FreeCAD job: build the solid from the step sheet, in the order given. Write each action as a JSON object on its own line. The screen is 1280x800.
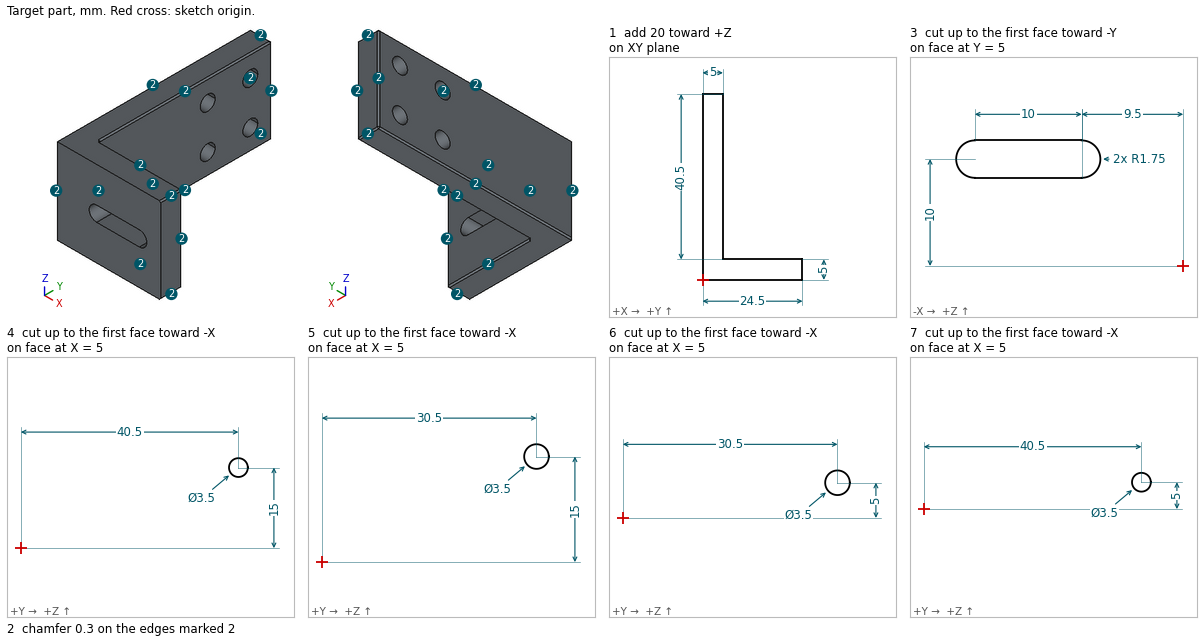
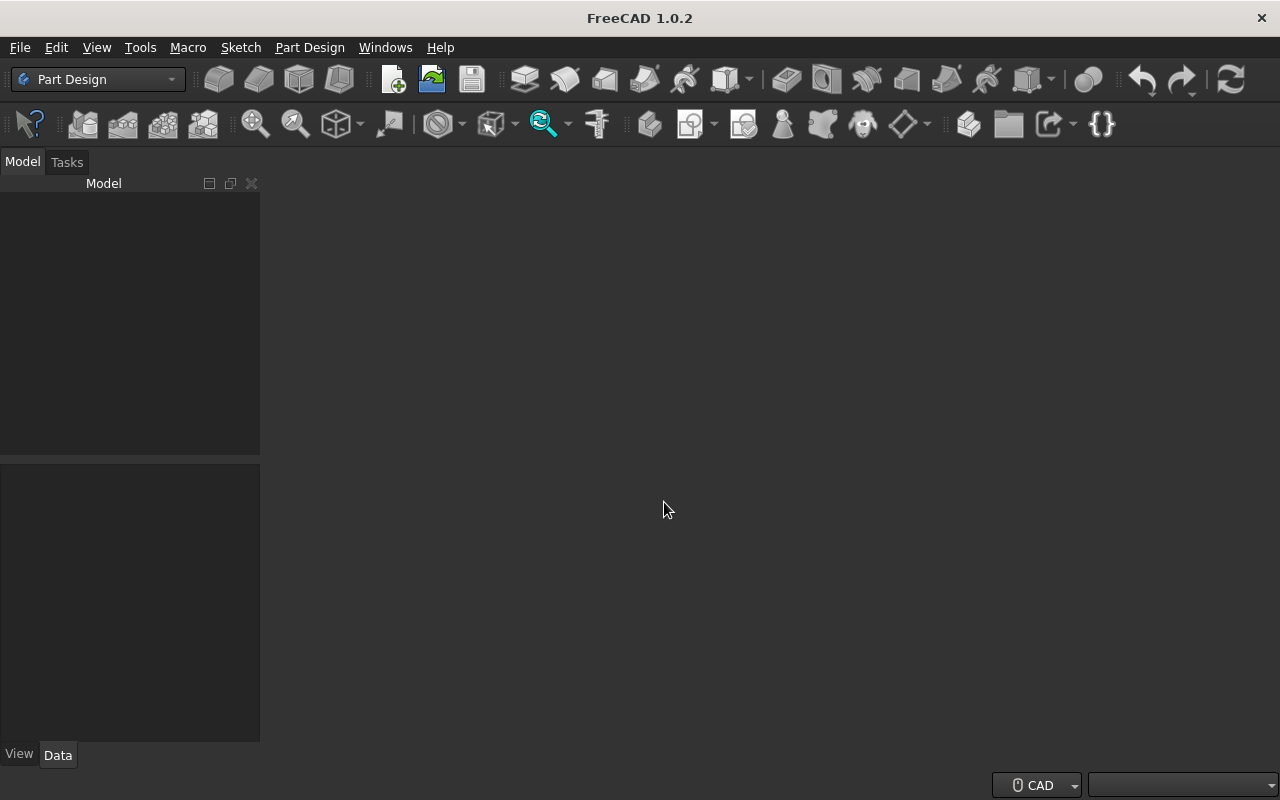
{"action": "left_click", "coordinate": [392, 80]}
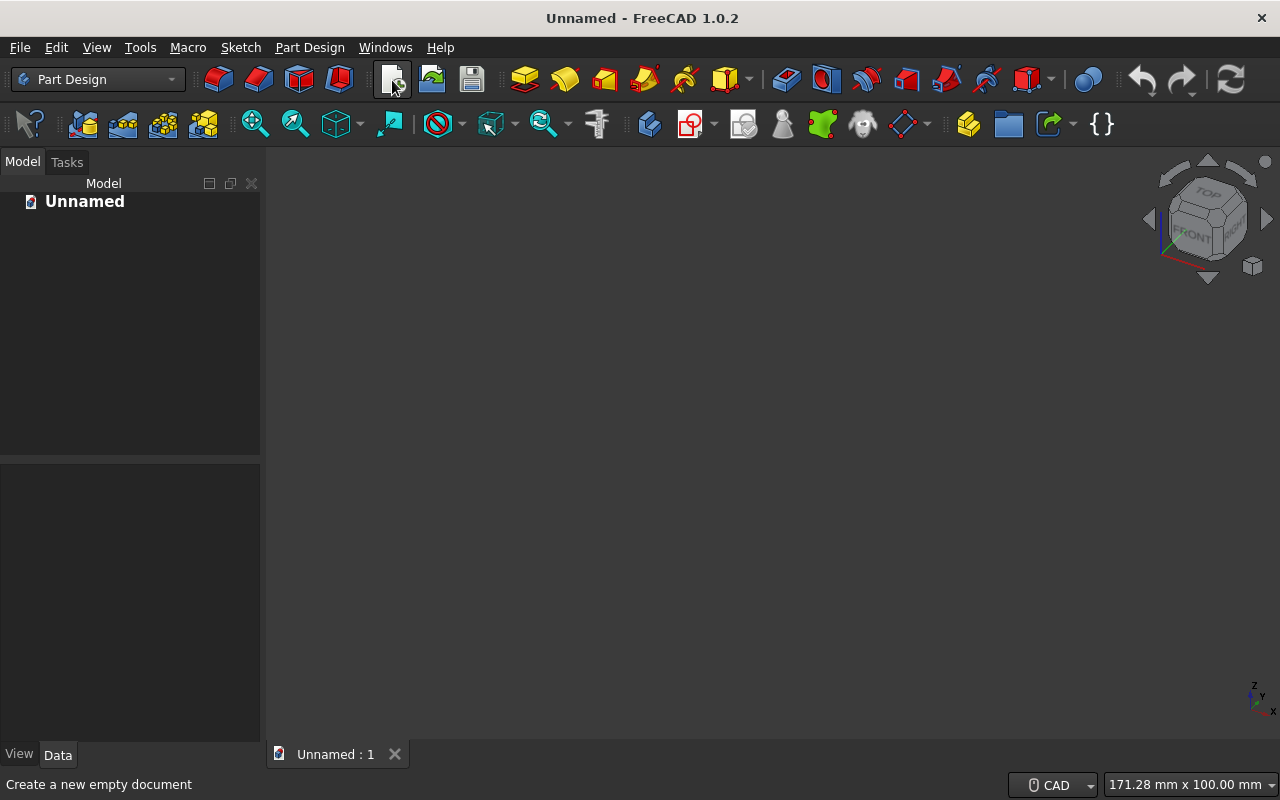
{"action": "left_click", "coordinate": [690, 124]}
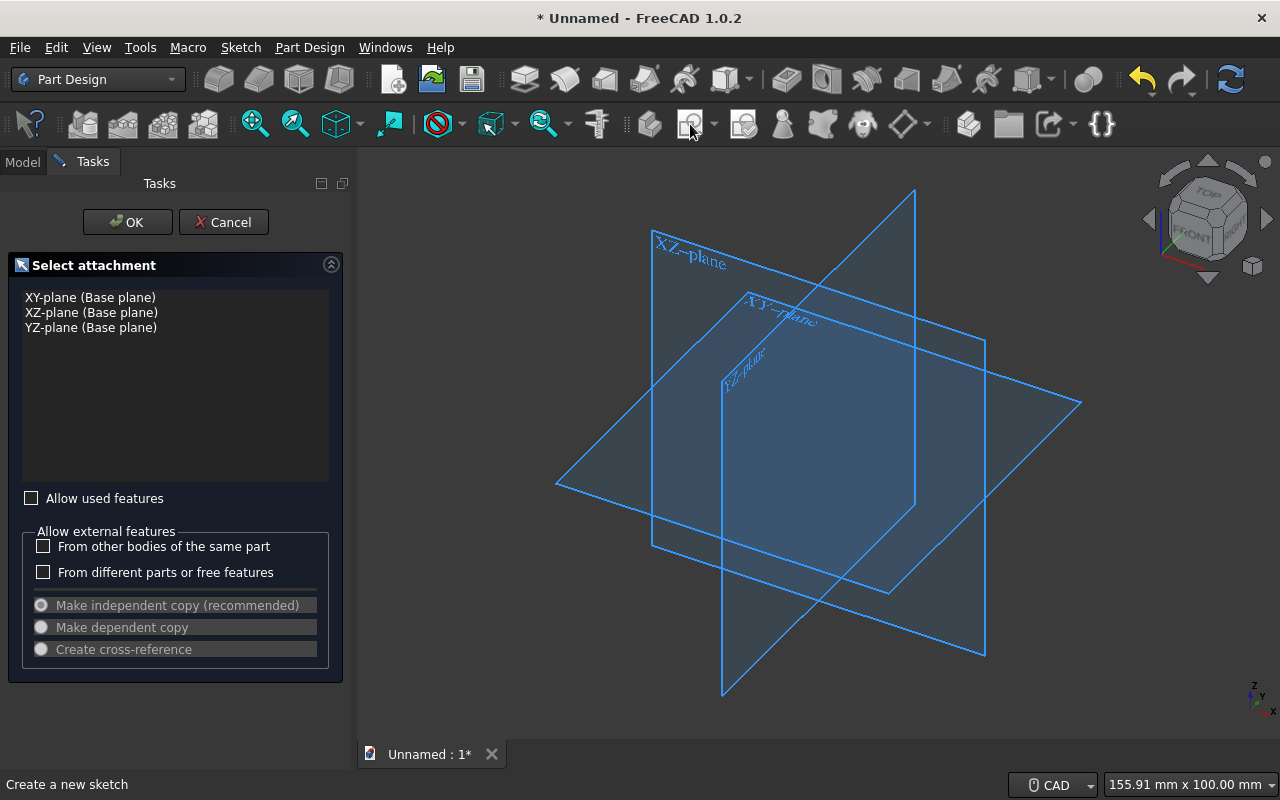
{"action": "left_click", "coordinate": [82, 298]}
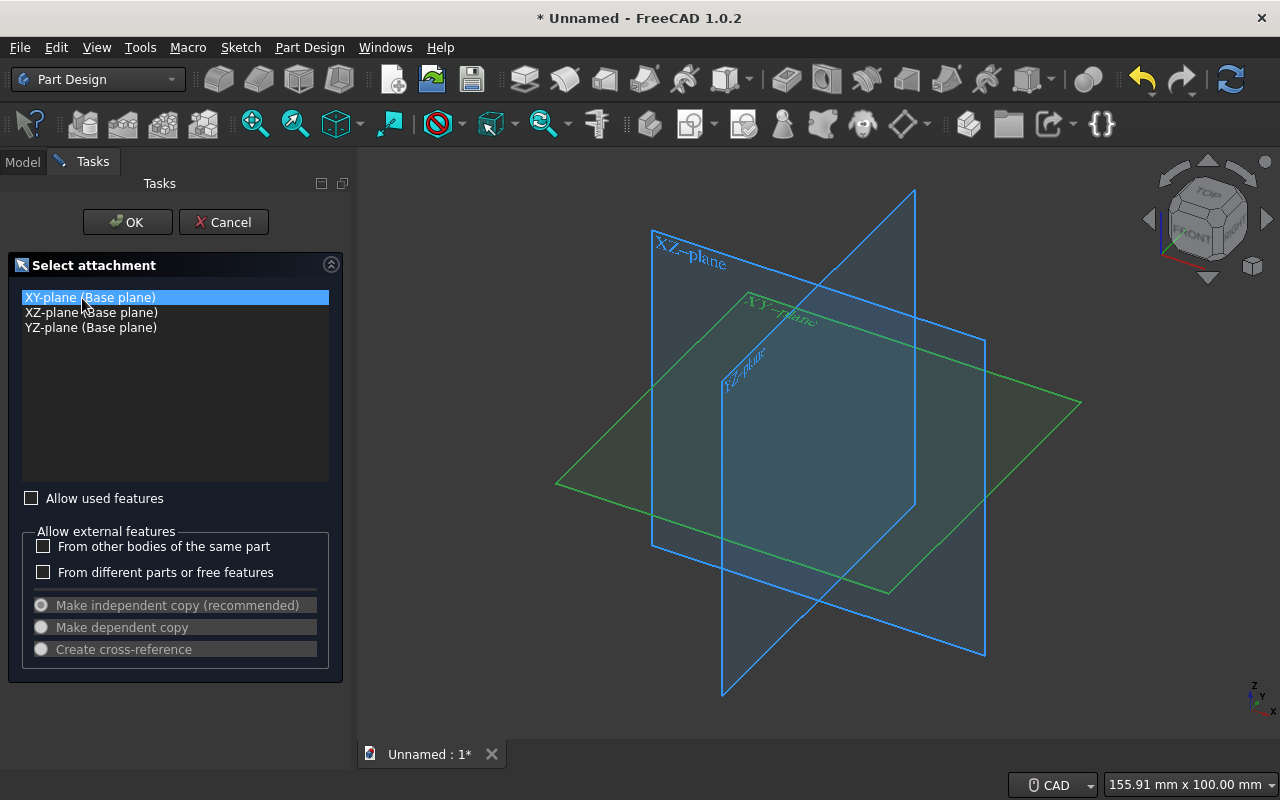
{"action": "left_click", "coordinate": [128, 222]}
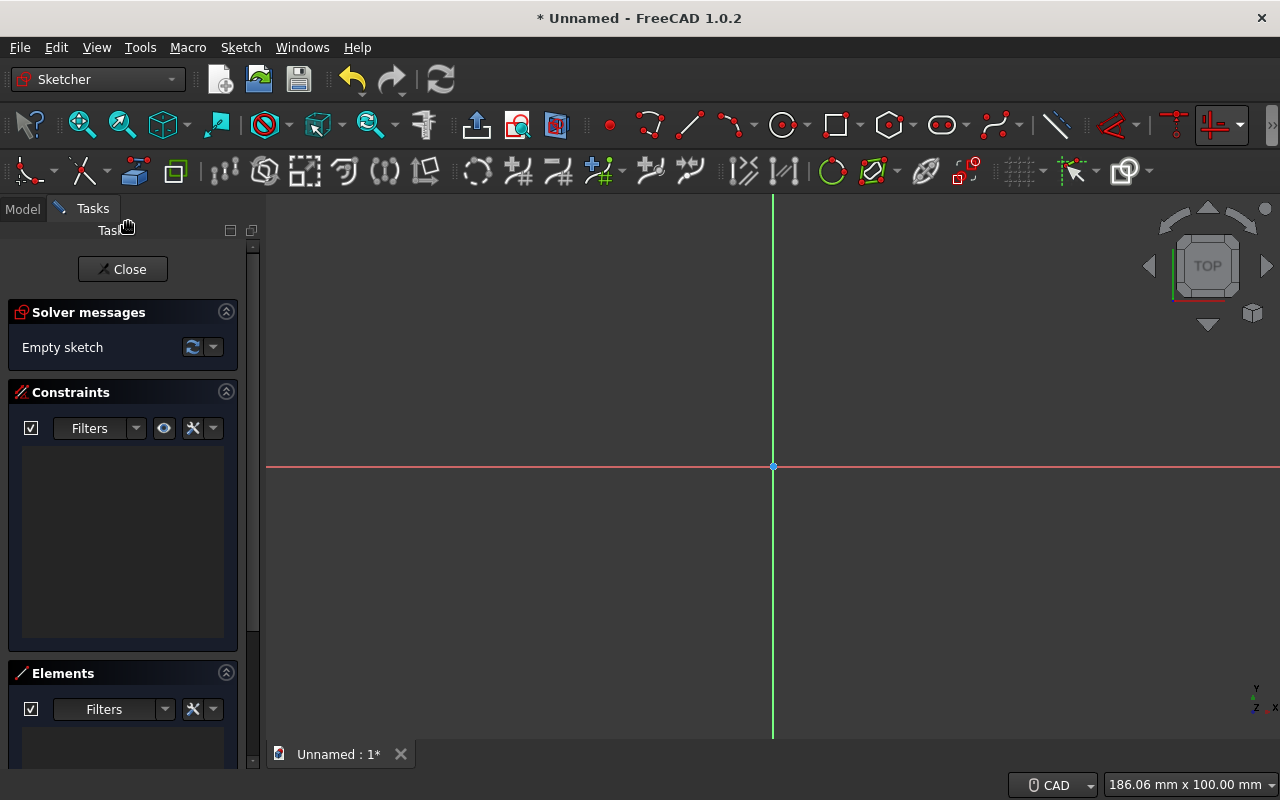
{"action": "scroll", "coordinate": [294, 711], "scroll_direction": "down", "scroll_amount": 1}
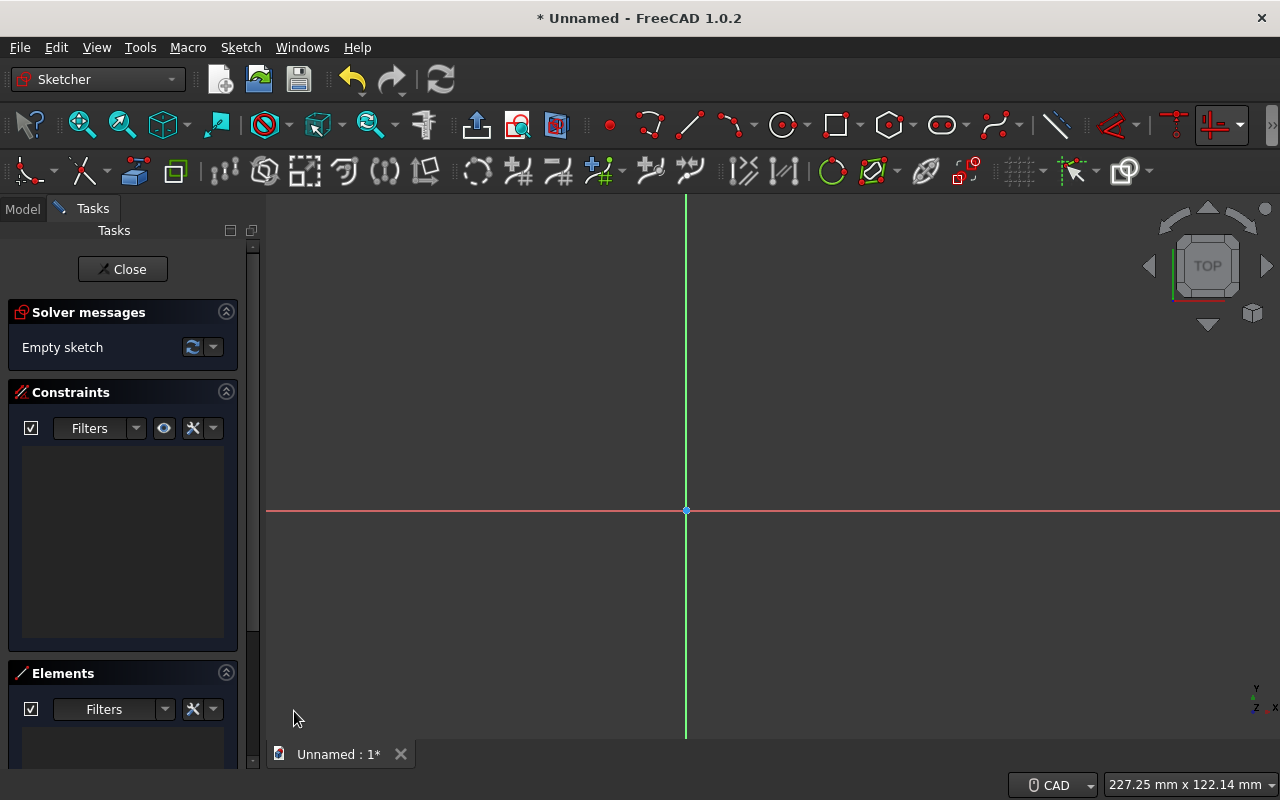
{"action": "scroll", "coordinate": [785, 340], "scroll_direction": "up", "scroll_amount": 3}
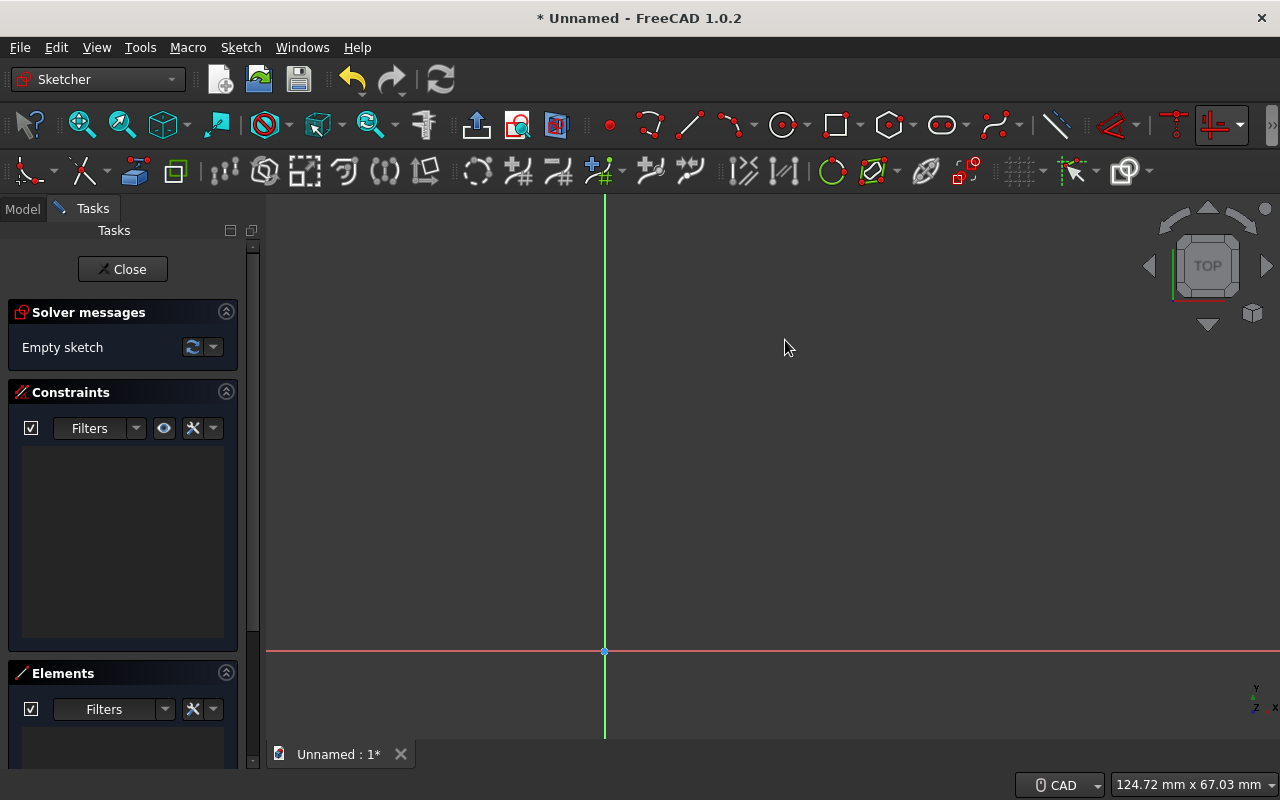
{"action": "key", "text": "g m"}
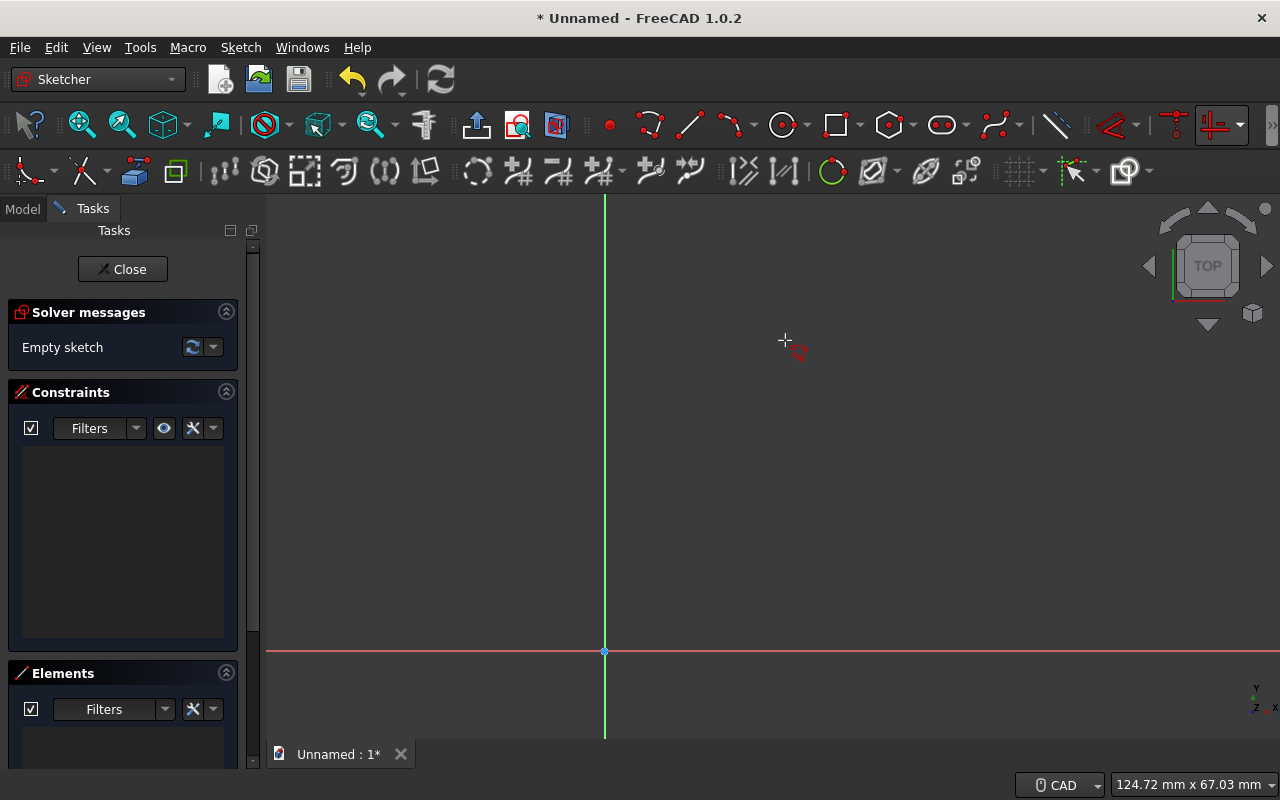
{"action": "left_click", "coordinate": [605, 651]}
{"action": "left_click", "coordinate": [804, 642]}
{"action": "left_click", "coordinate": [804, 611]}
{"action": "left_click", "coordinate": [645, 611]}
{"action": "left_click", "coordinate": [645, 281]}
{"action": "left_click", "coordinate": [614, 281]}
{"action": "left_click", "coordinate": [605, 651]}
{"action": "key", "text": "Escape"}
{"action": "key", "text": "Escape"}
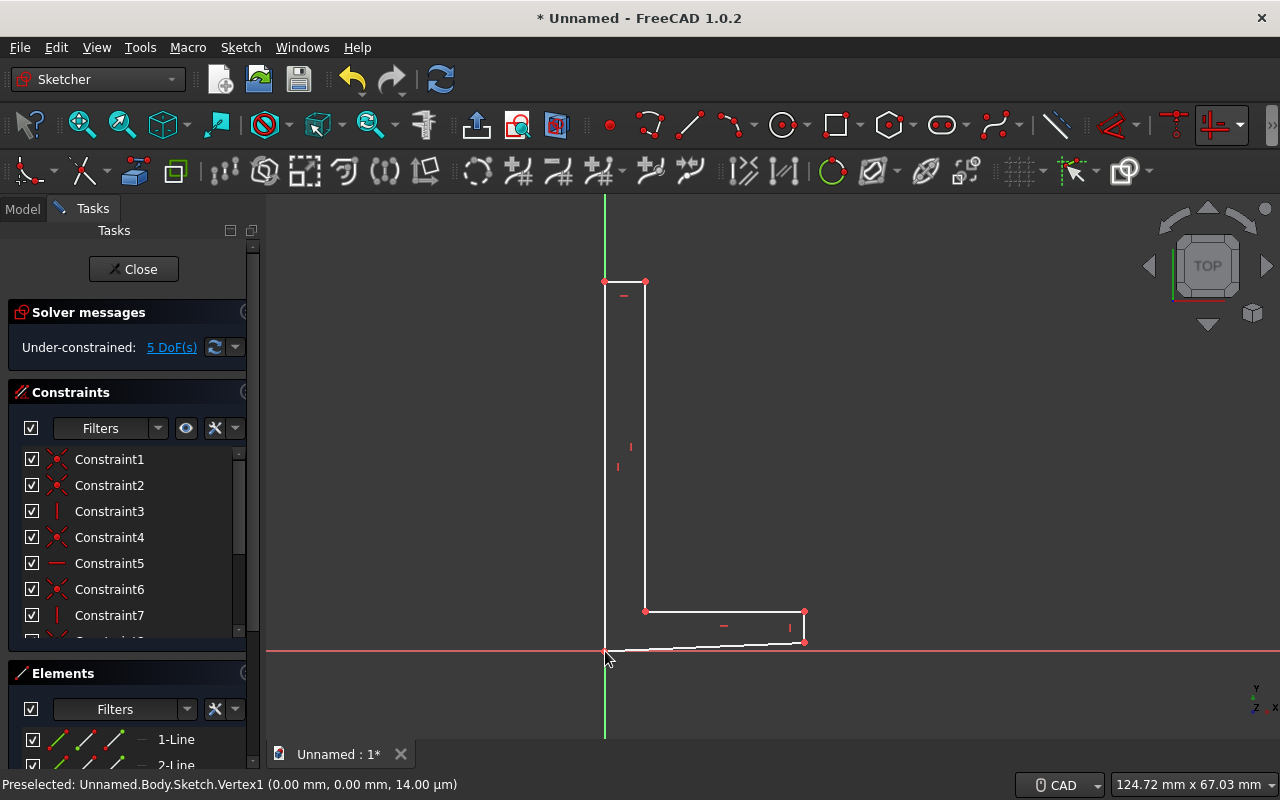
{"action": "left_click", "coordinate": [664, 649]}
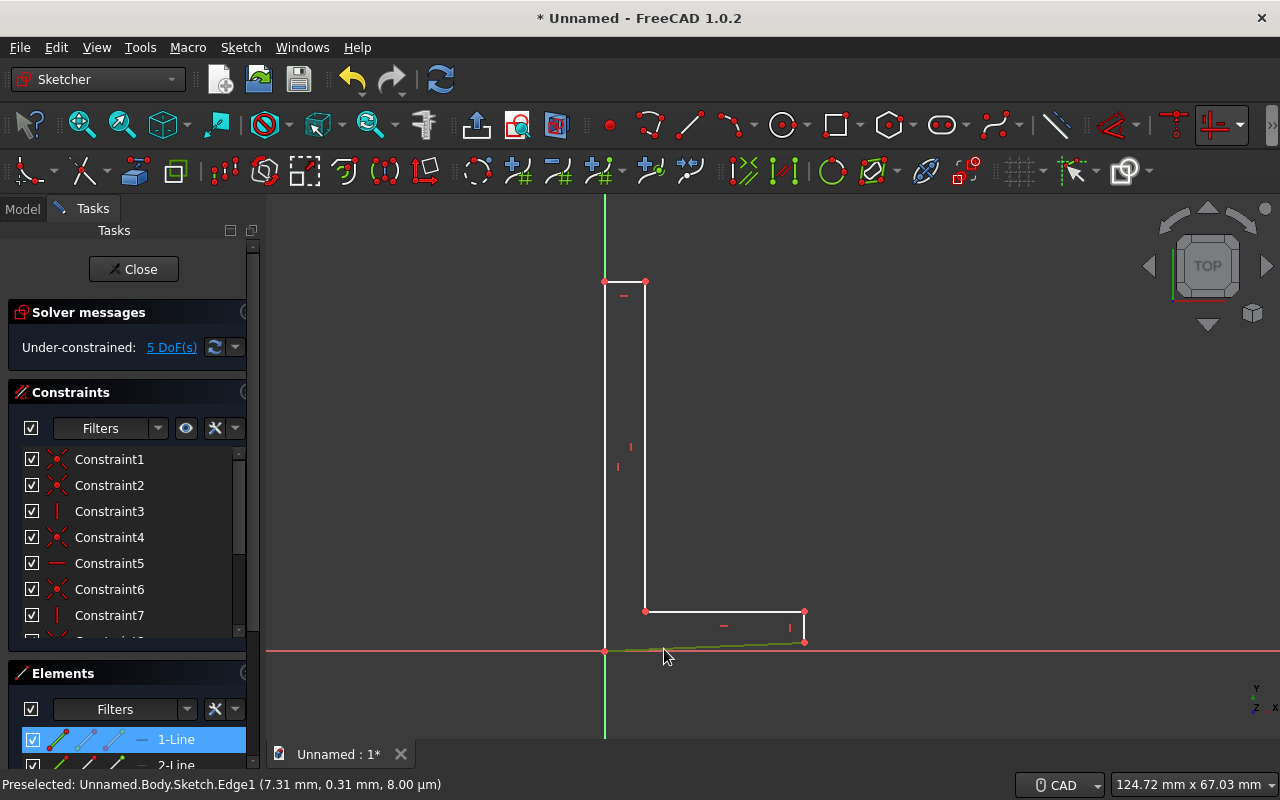
{"action": "left_click", "coordinate": [1242, 126]}